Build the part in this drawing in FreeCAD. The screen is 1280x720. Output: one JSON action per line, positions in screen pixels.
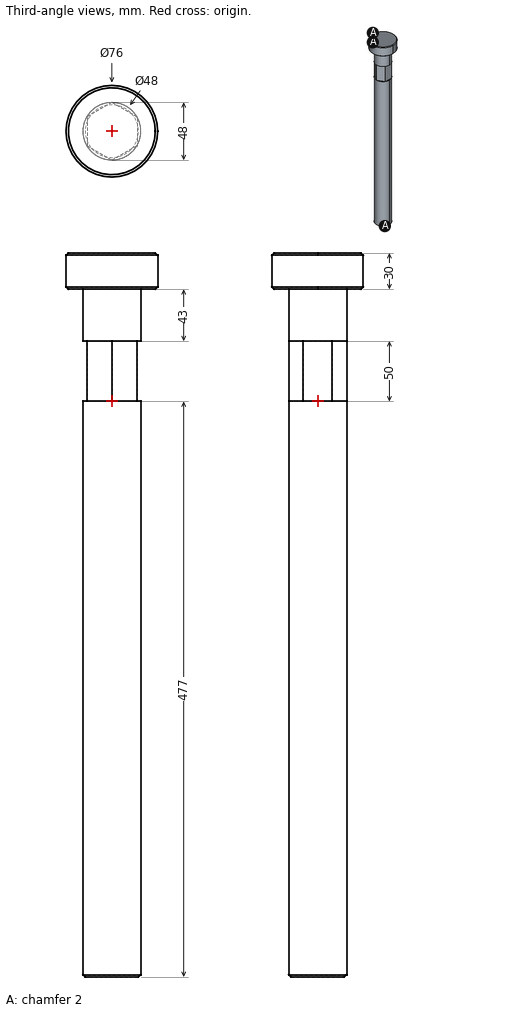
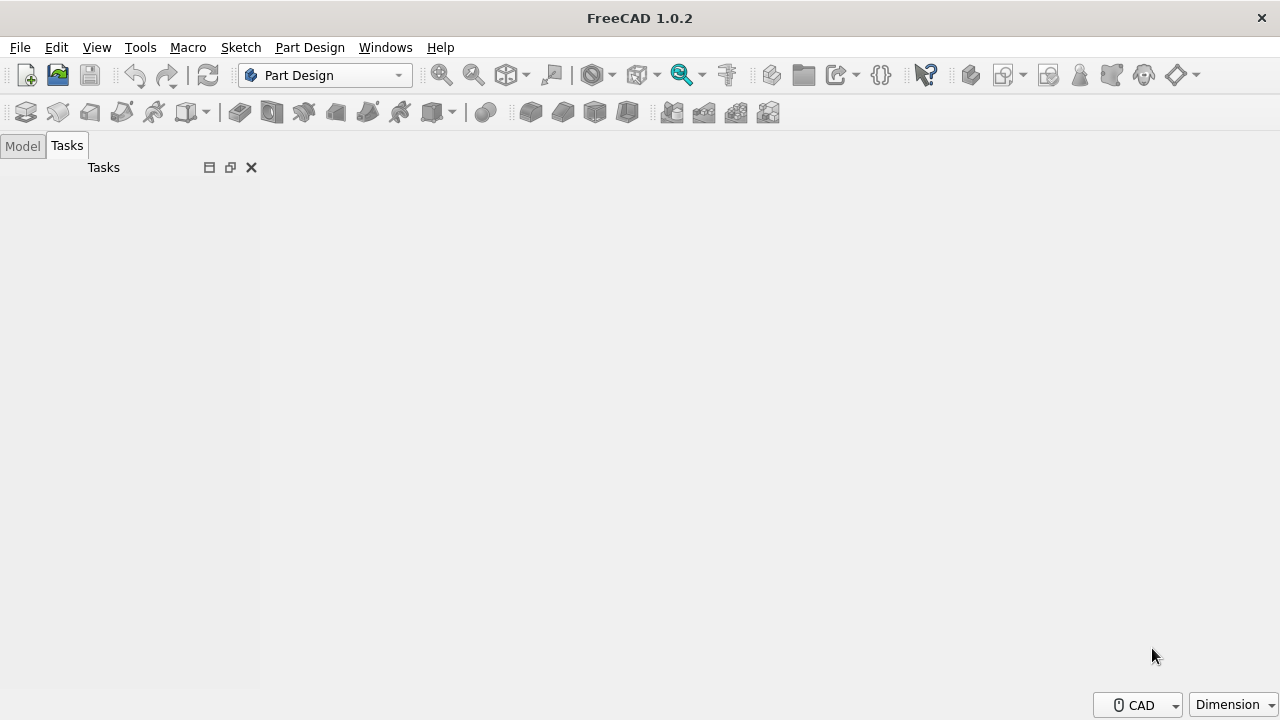
{"action": "left_click", "coordinate": [26, 76]}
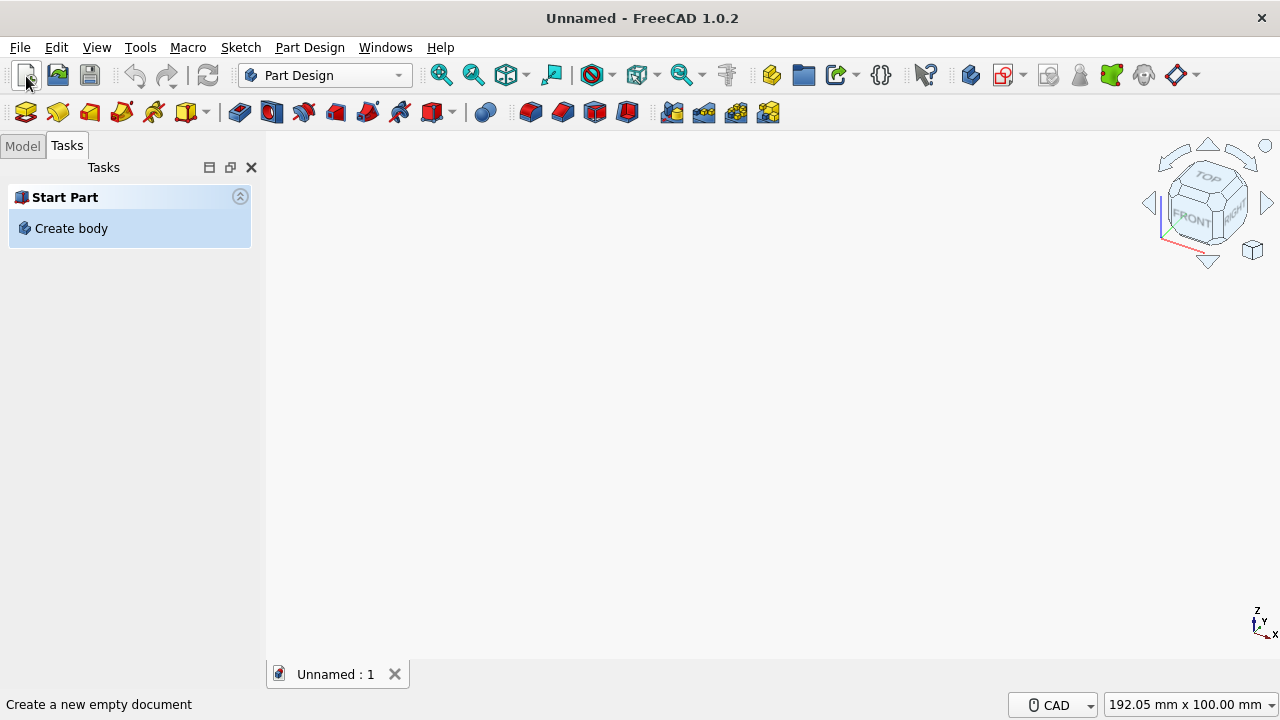
{"action": "left_click", "coordinate": [1004, 76]}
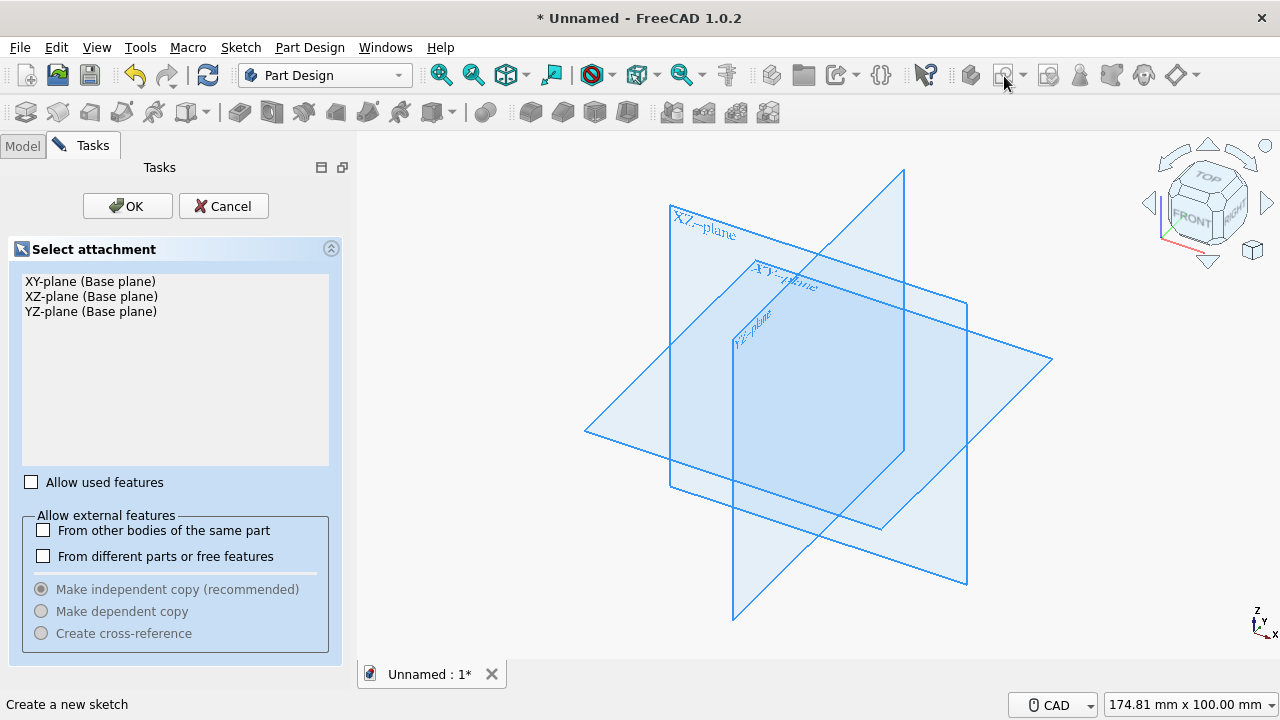
{"action": "left_click", "coordinate": [82, 282]}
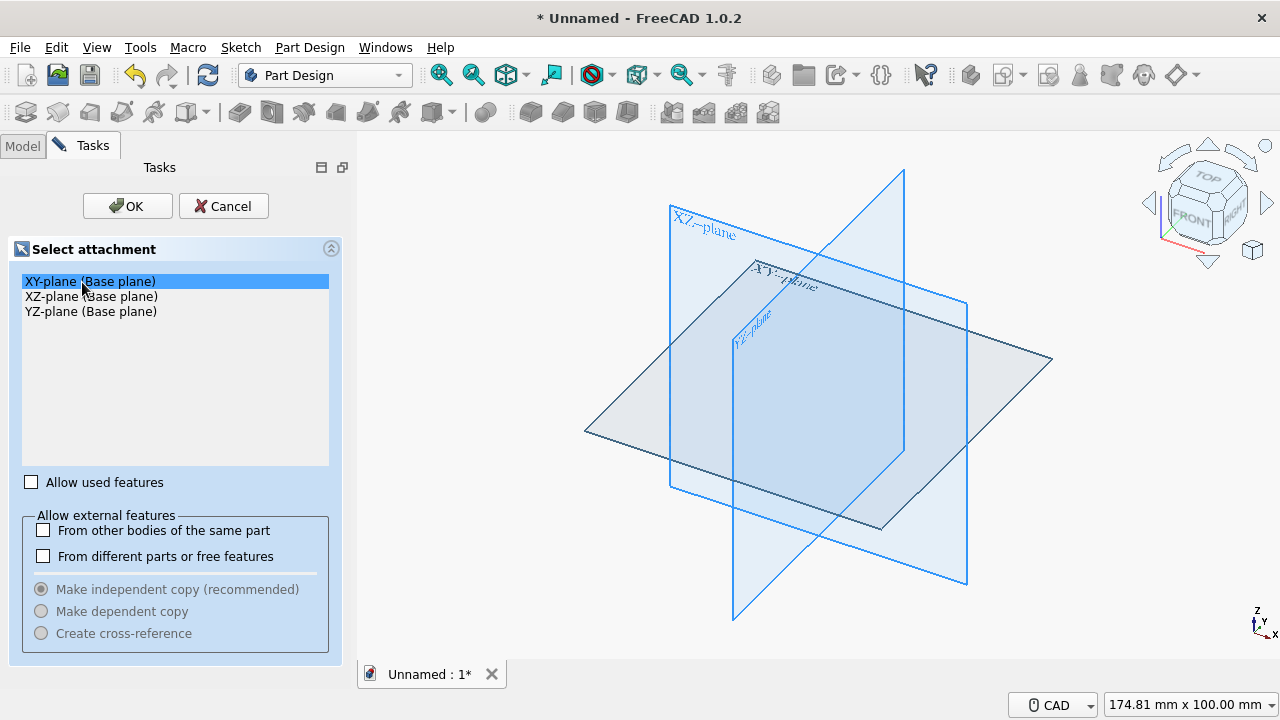
{"action": "left_click", "coordinate": [128, 206]}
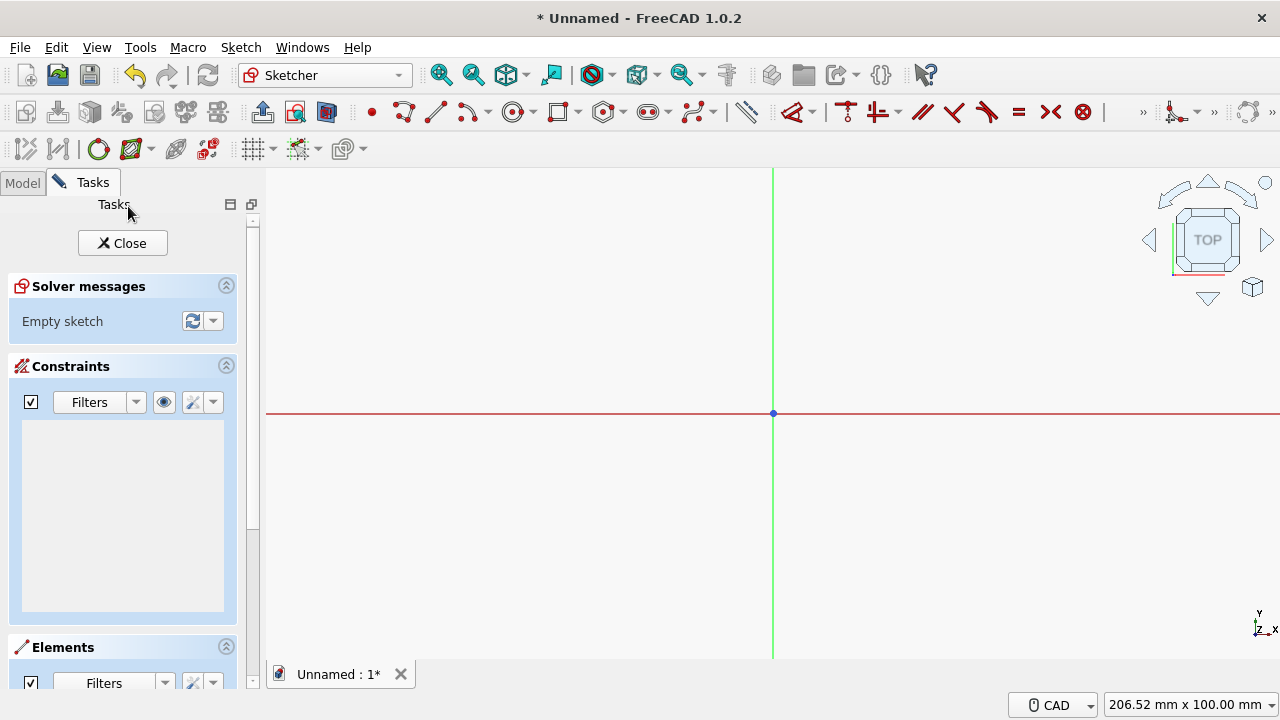
{"action": "left_click", "coordinate": [604, 112]}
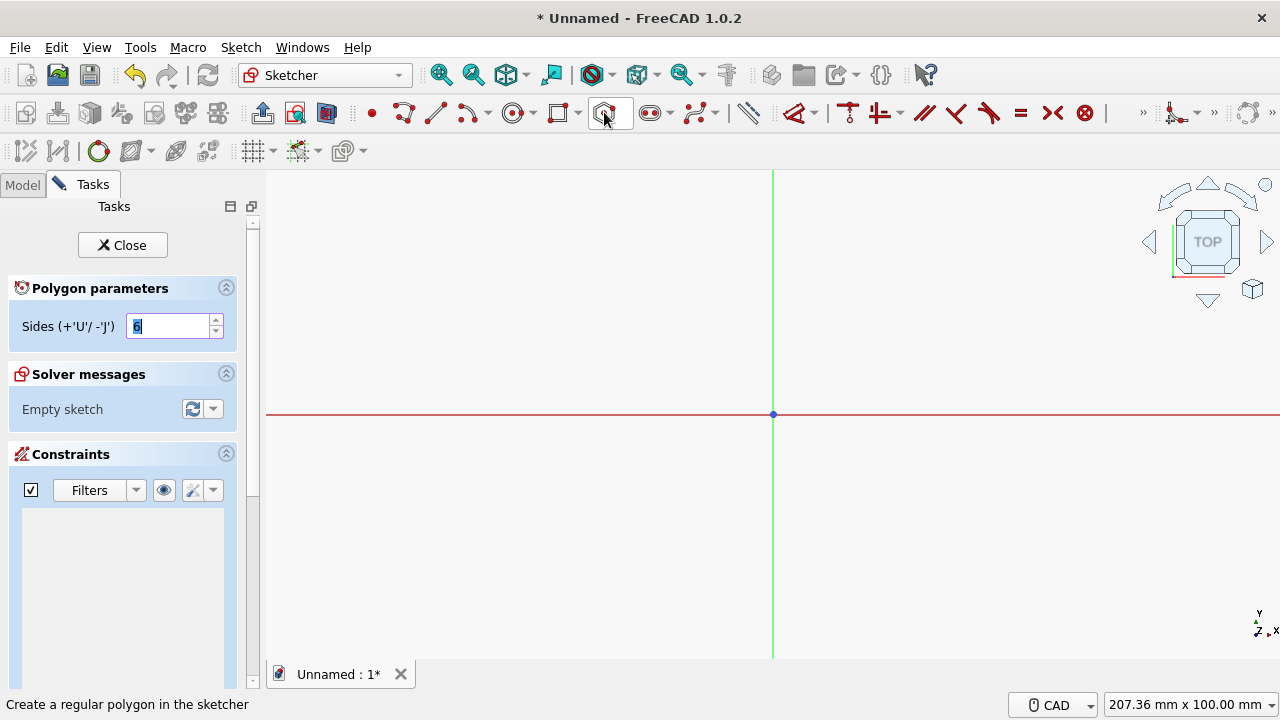
{"action": "left_click", "coordinate": [773, 414]}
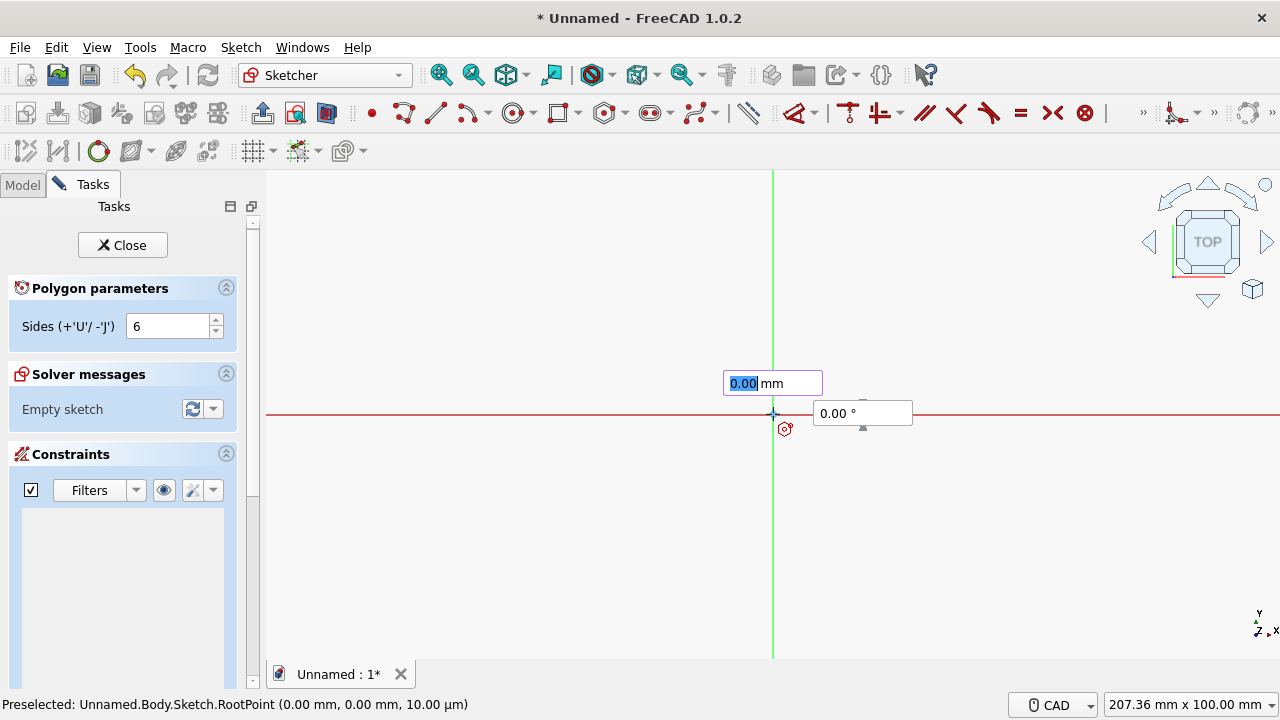
{"action": "left_click", "coordinate": [773, 297]}
{"action": "right_click", "coordinate": [773, 297]}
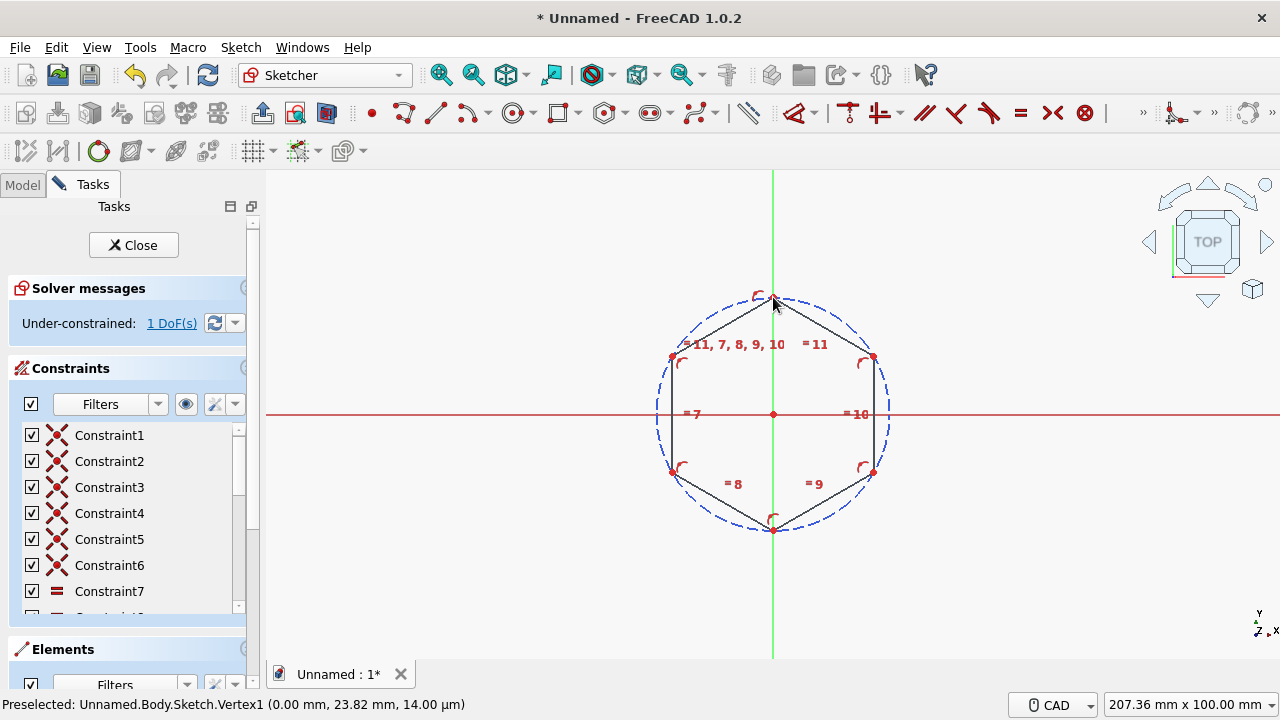
{"action": "left_click", "coordinate": [794, 114]}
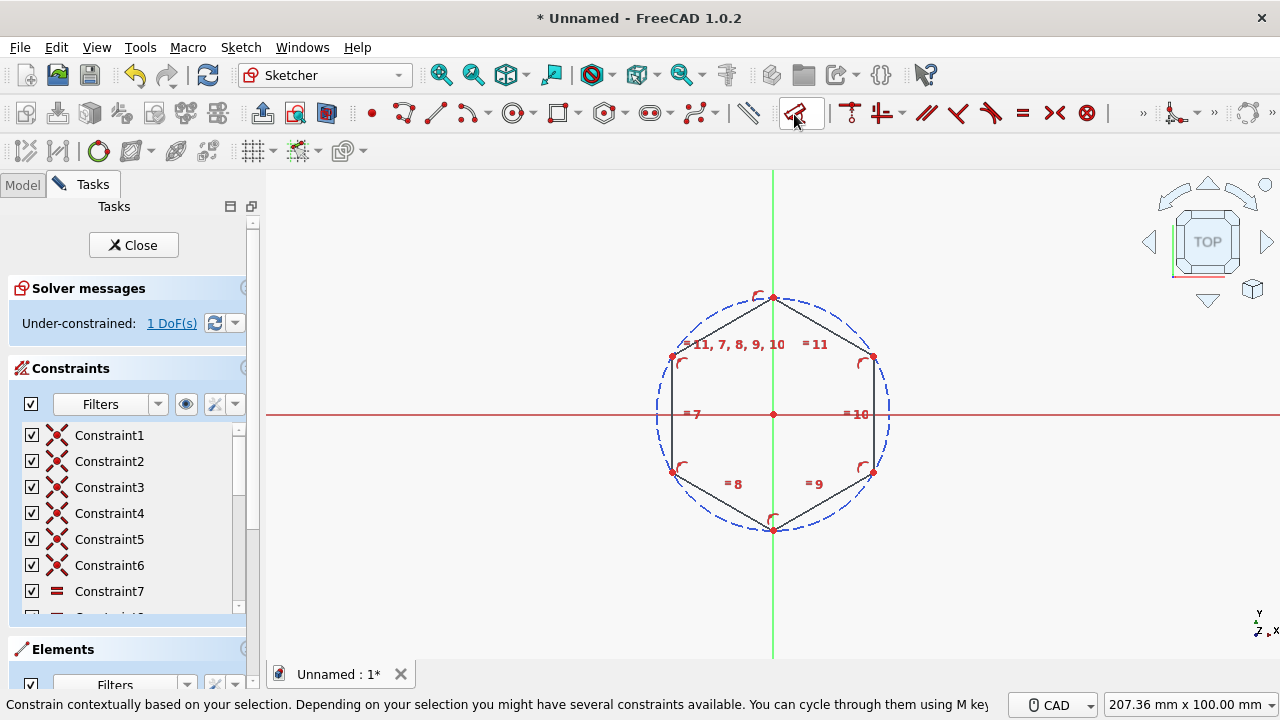
{"action": "left_click", "coordinate": [773, 531]}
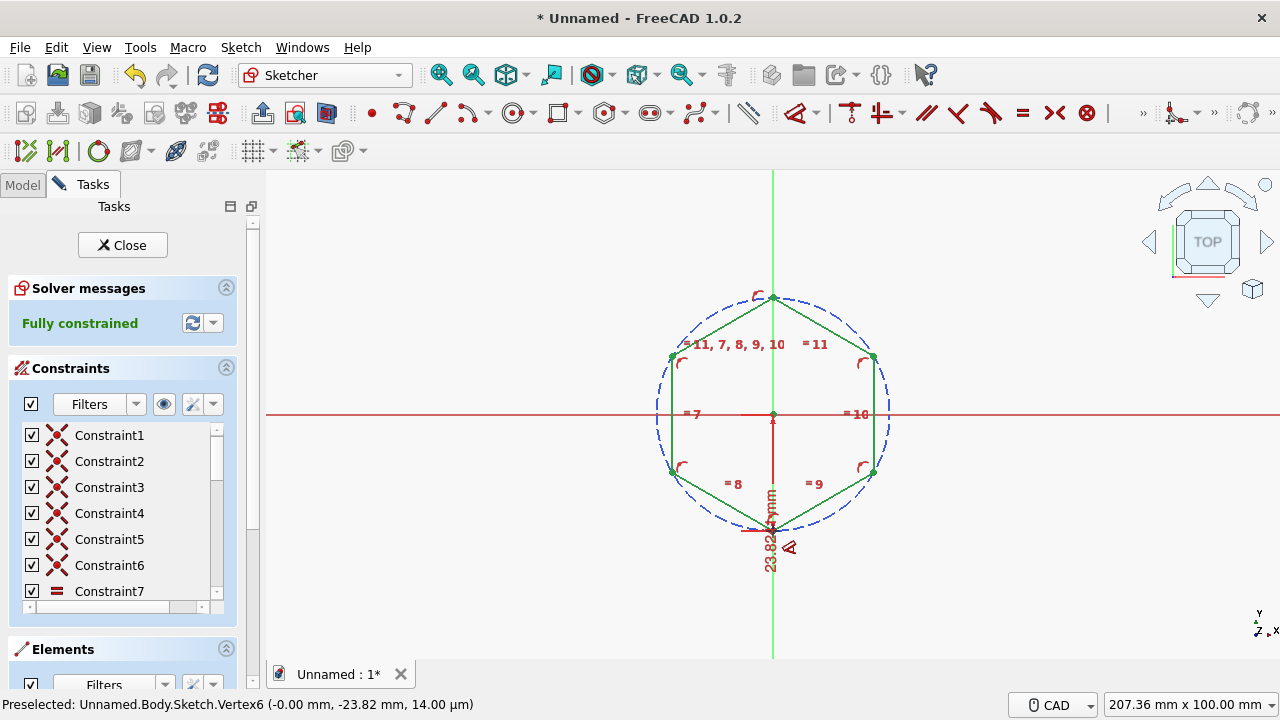
{"action": "left_click", "coordinate": [773, 298]}
{"action": "left_click", "coordinate": [807, 361]}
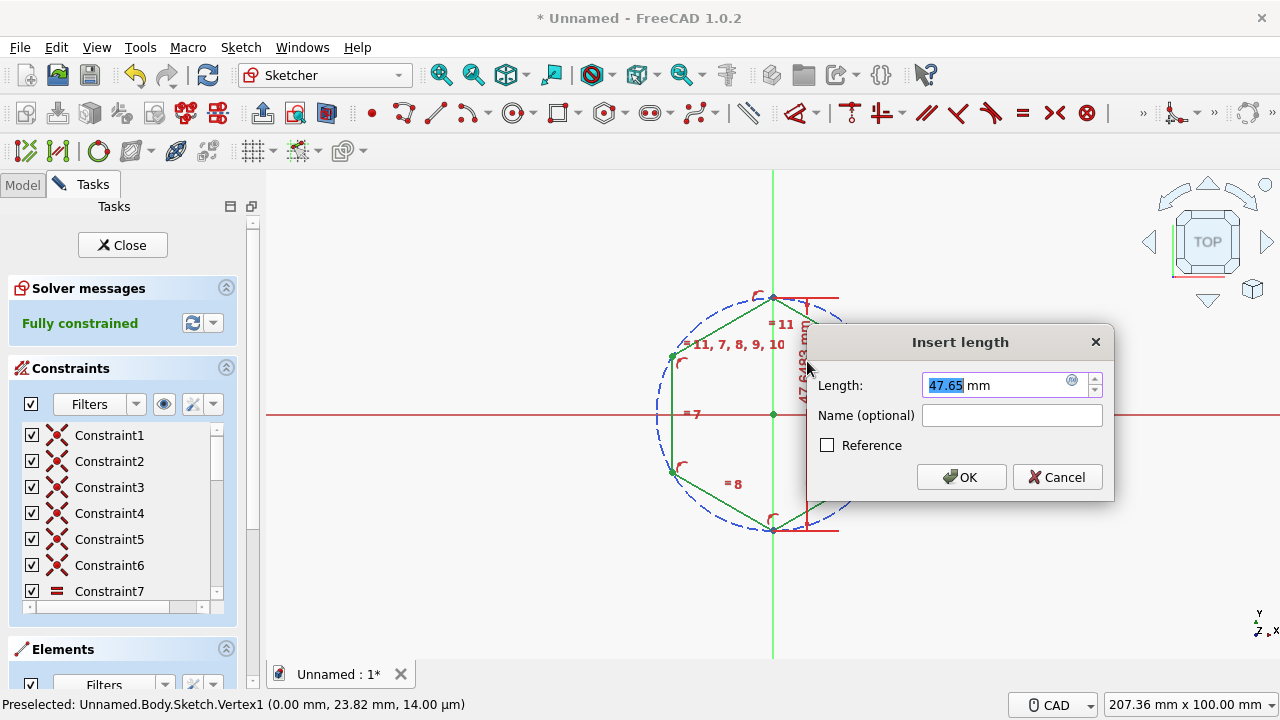
{"action": "type", "text": "48"}
{"action": "key", "text": "Return"}
{"action": "key", "text": "Escape"}